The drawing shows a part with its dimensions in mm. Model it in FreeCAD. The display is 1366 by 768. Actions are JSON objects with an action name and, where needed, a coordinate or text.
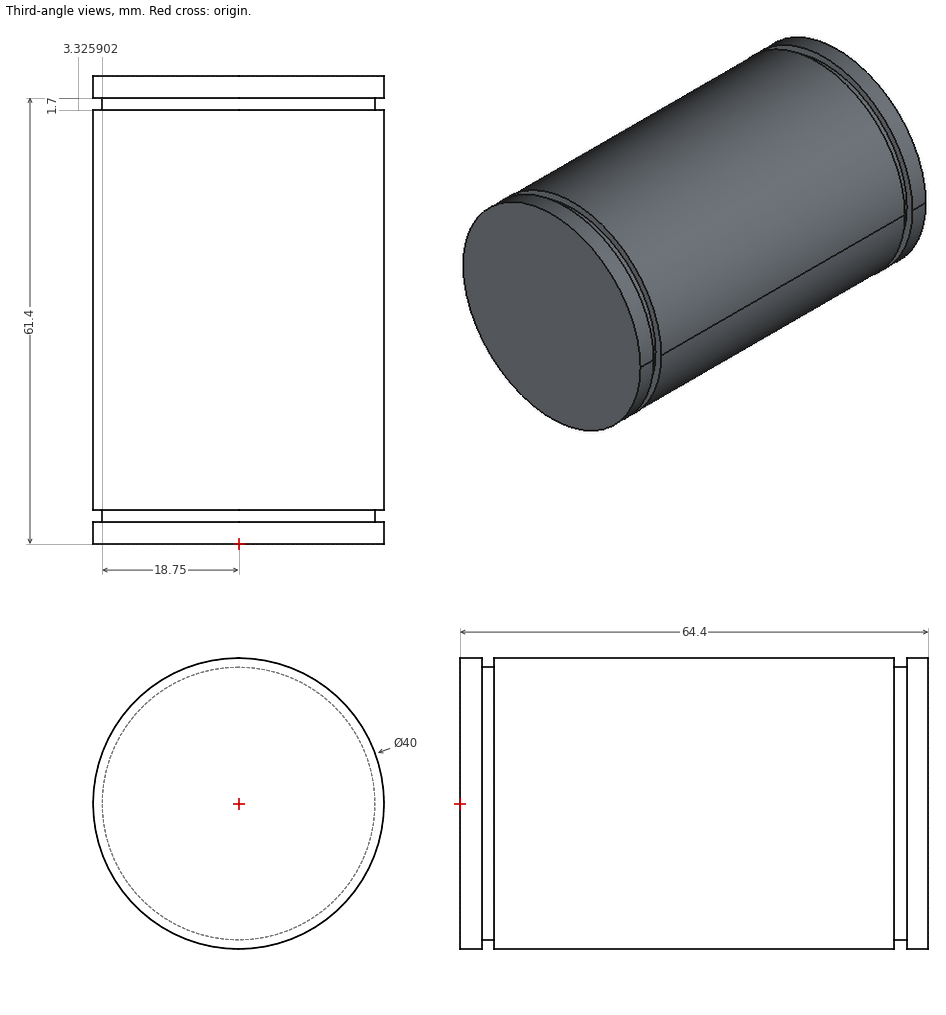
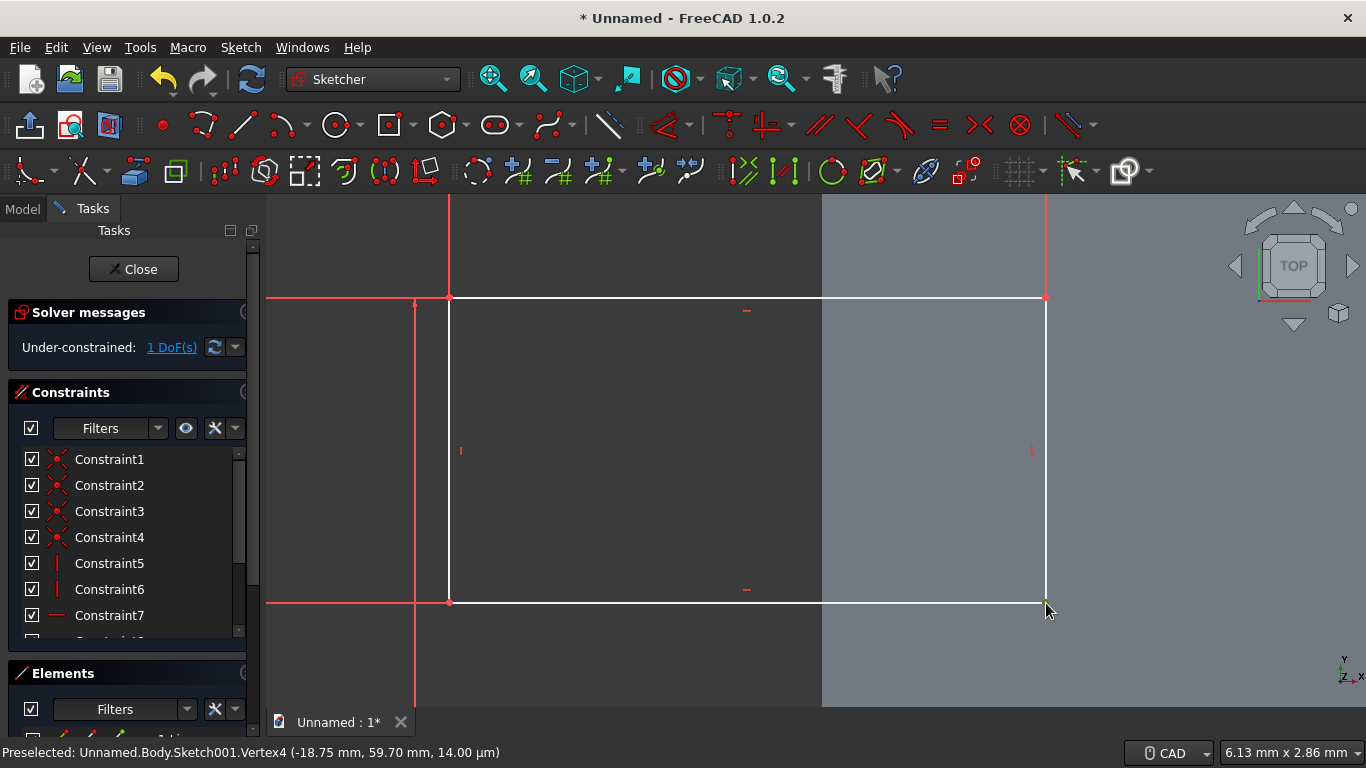
{"action": "left_click", "coordinate": [692, 126]}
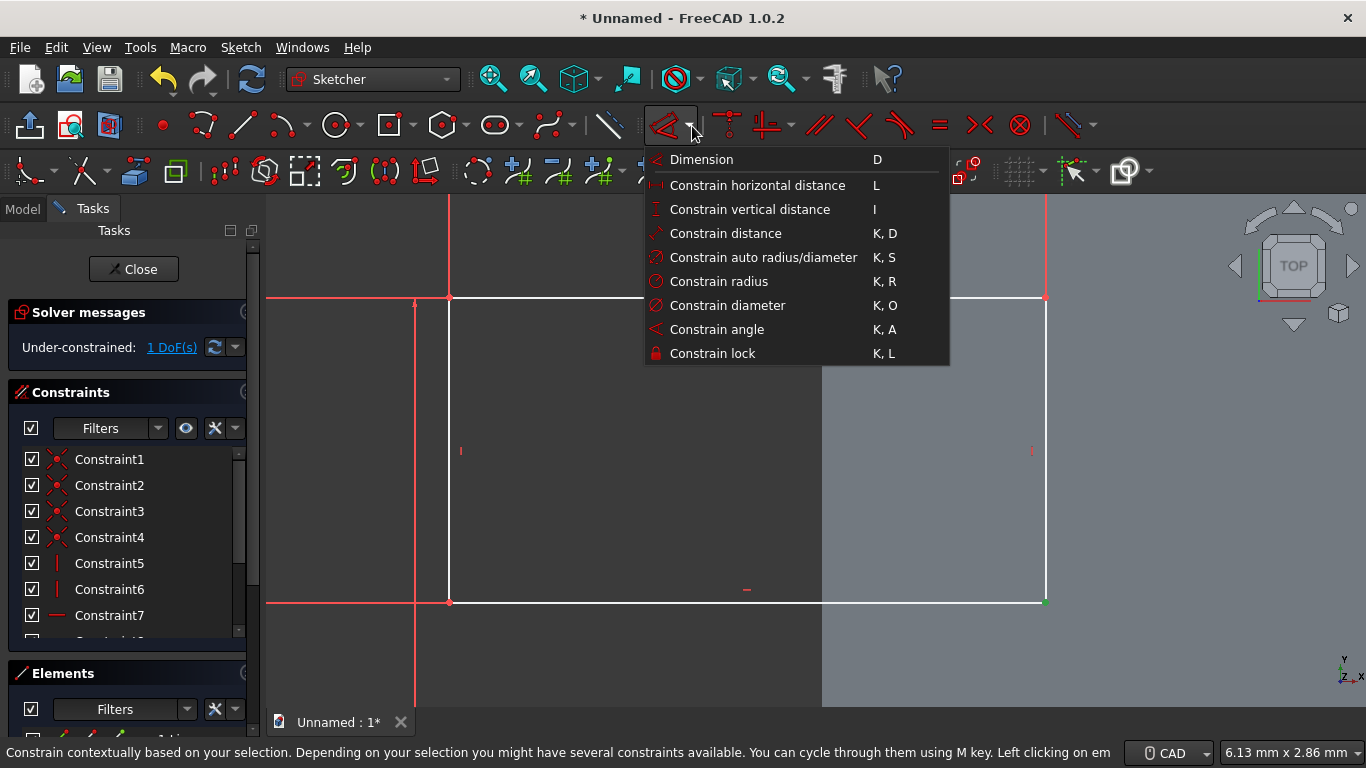
{"action": "left_click", "coordinate": [797, 185]}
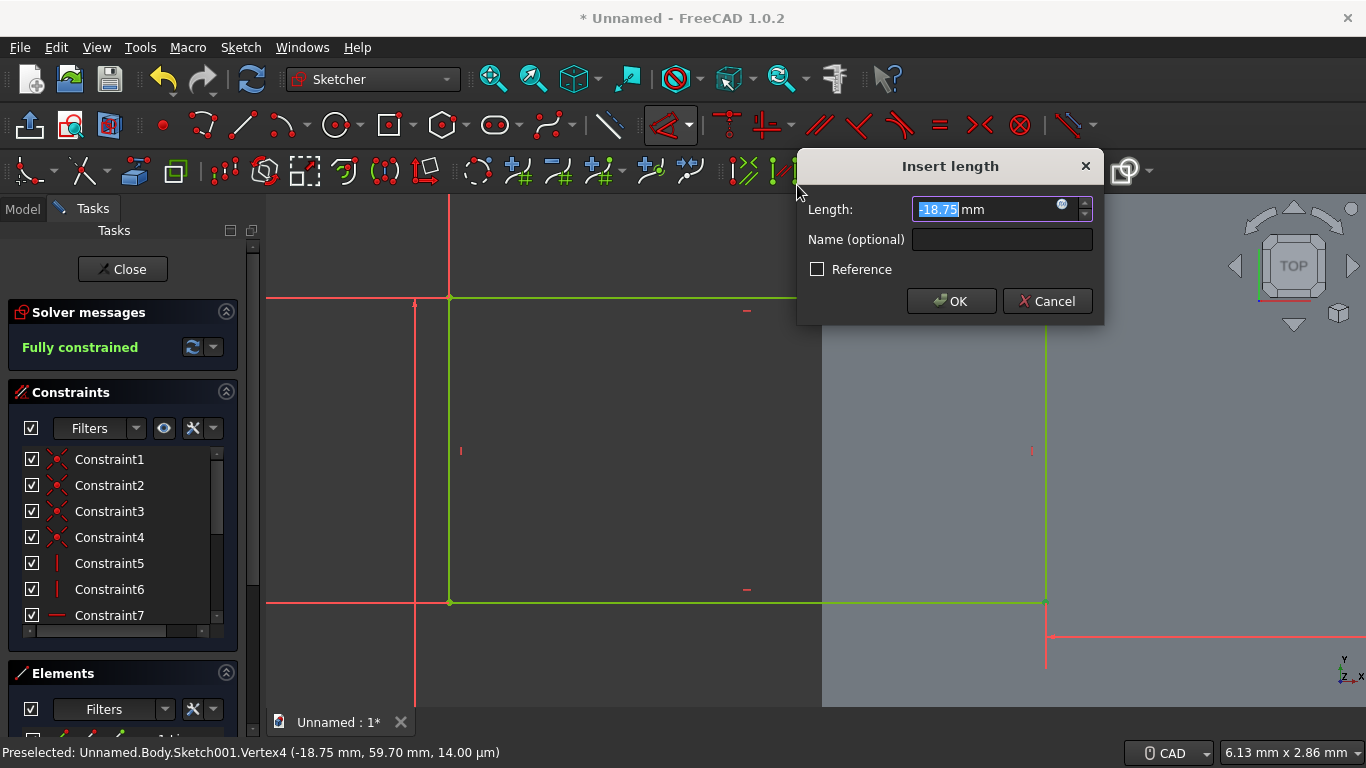
{"action": "type", "text": "-18.75"}
{"action": "key", "text": "Return"}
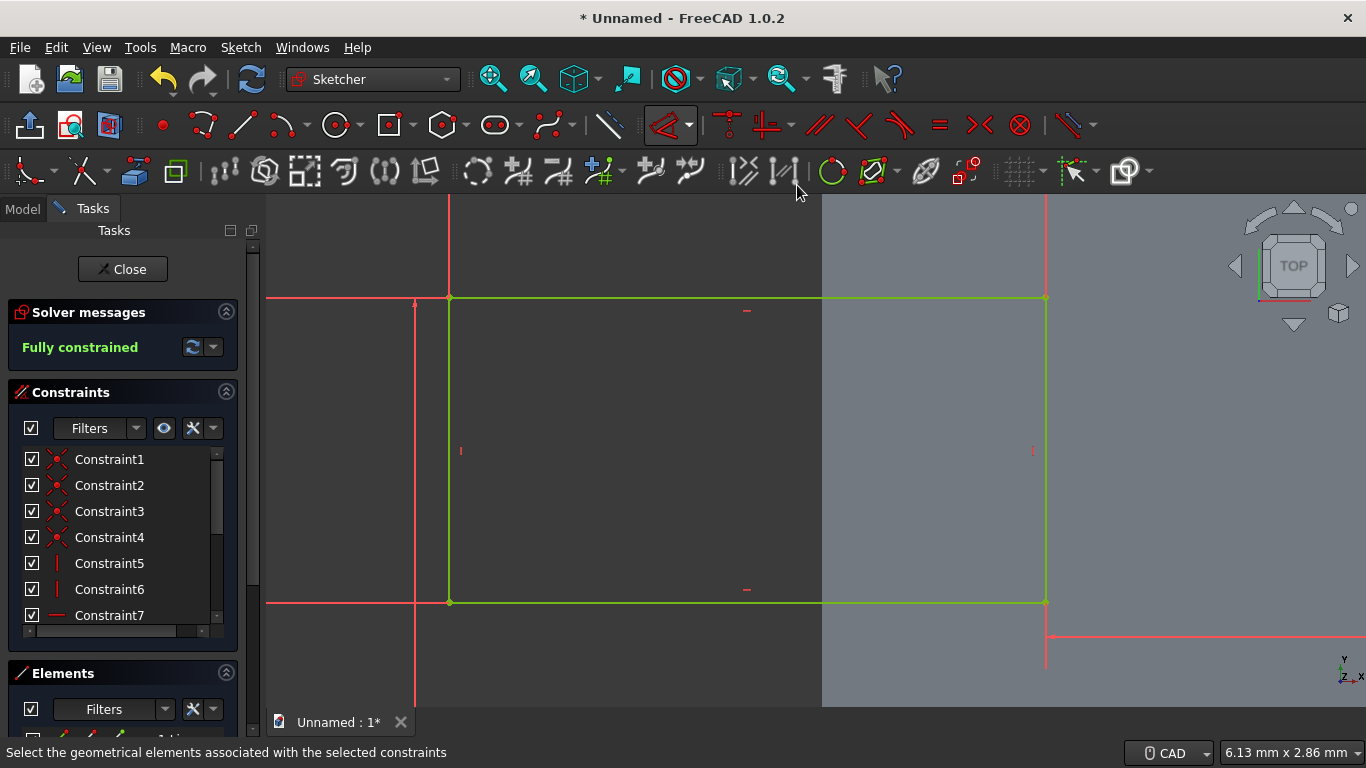
{"action": "left_click", "coordinate": [123, 269]}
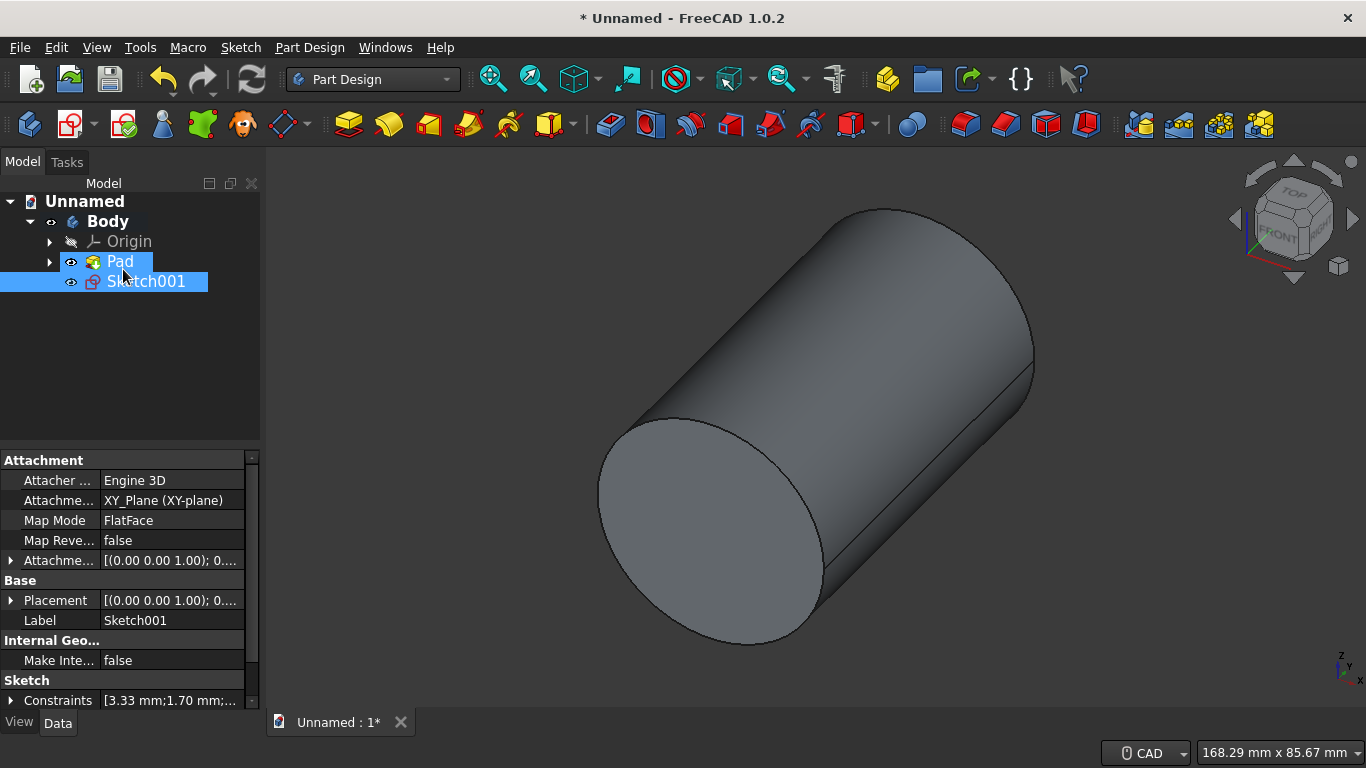
{"action": "left_click", "coordinate": [692, 124]}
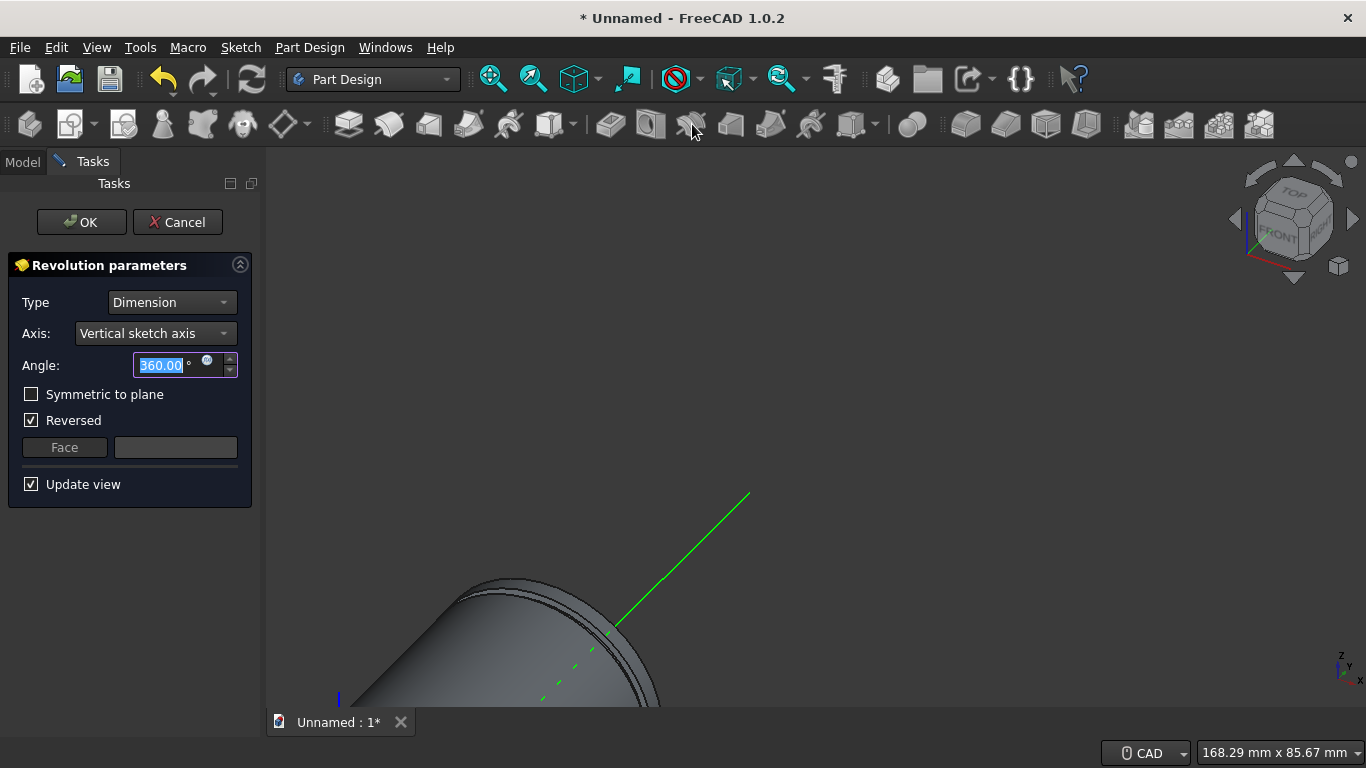
{"action": "left_click", "coordinate": [82, 222]}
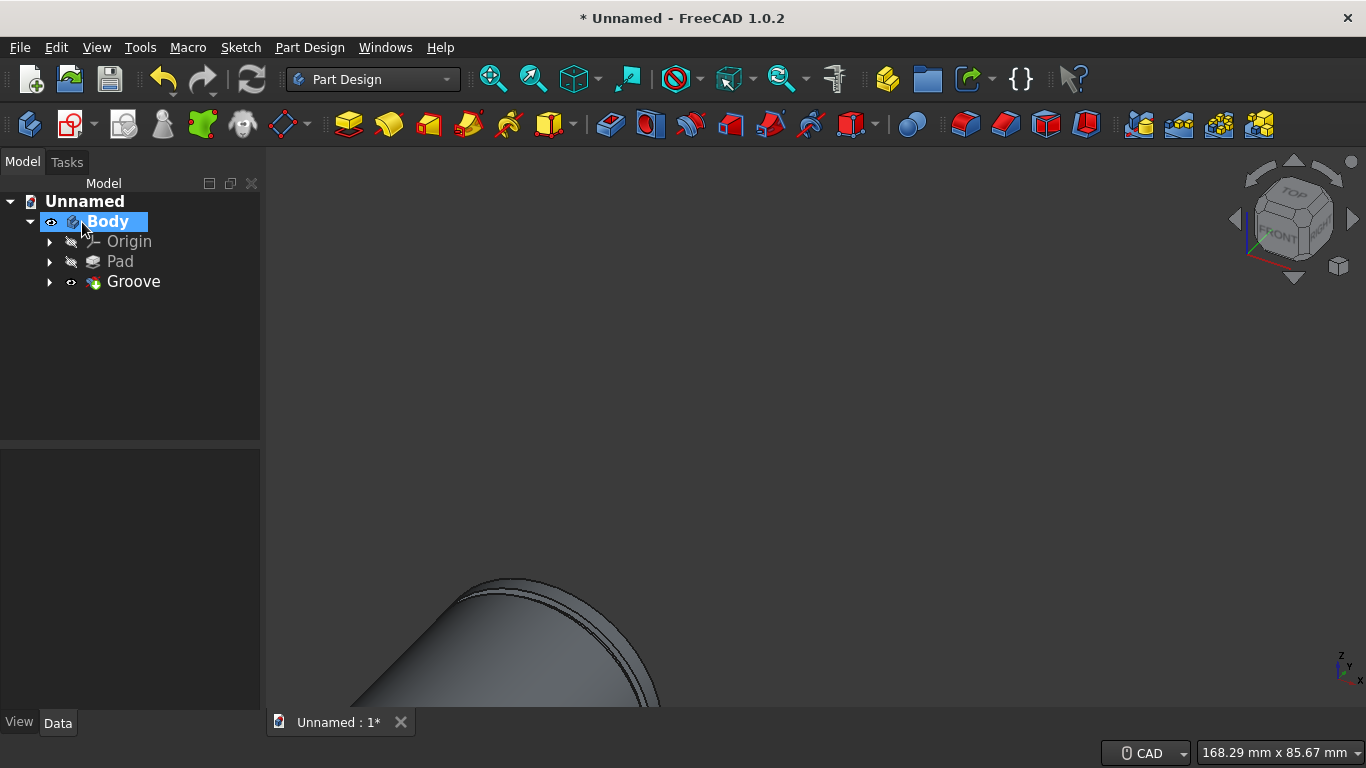
{"action": "left_click", "coordinate": [494, 80]}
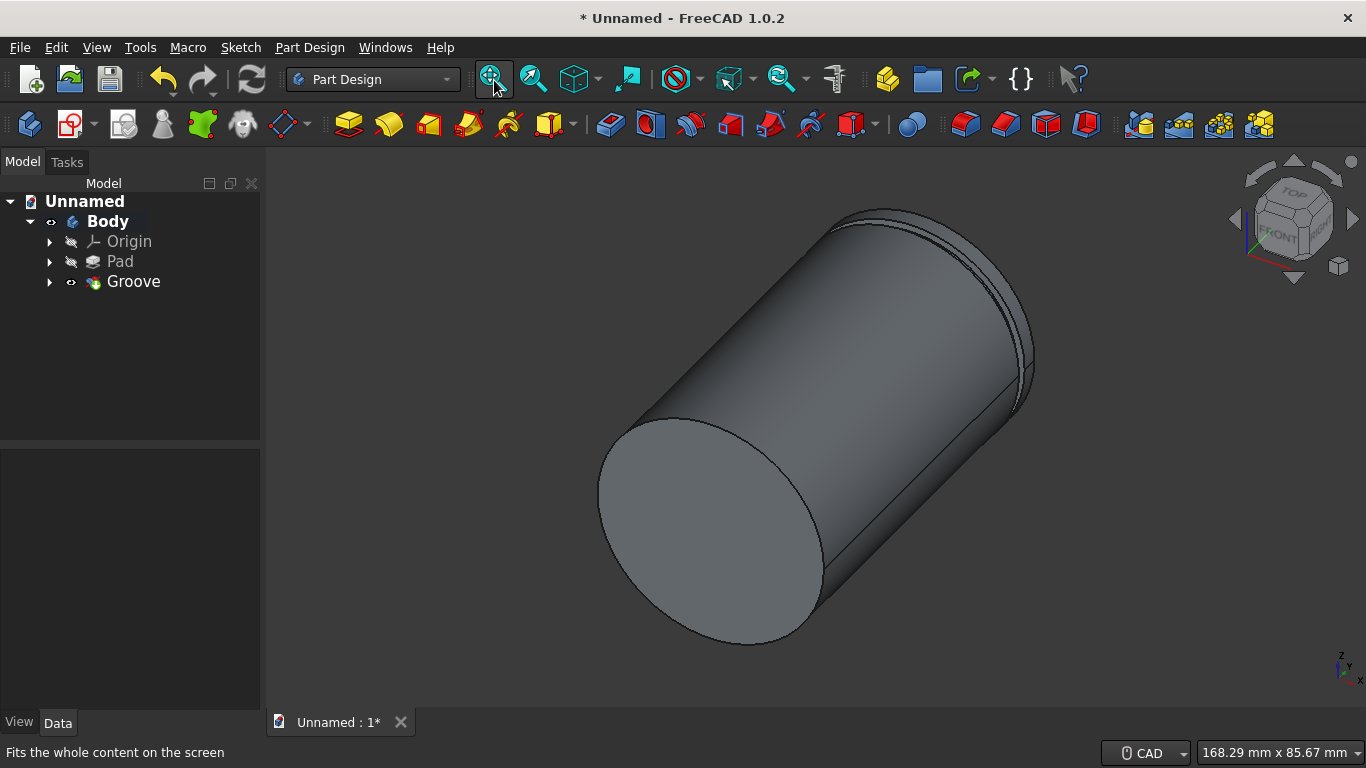
{"action": "left_click", "coordinate": [50, 242]}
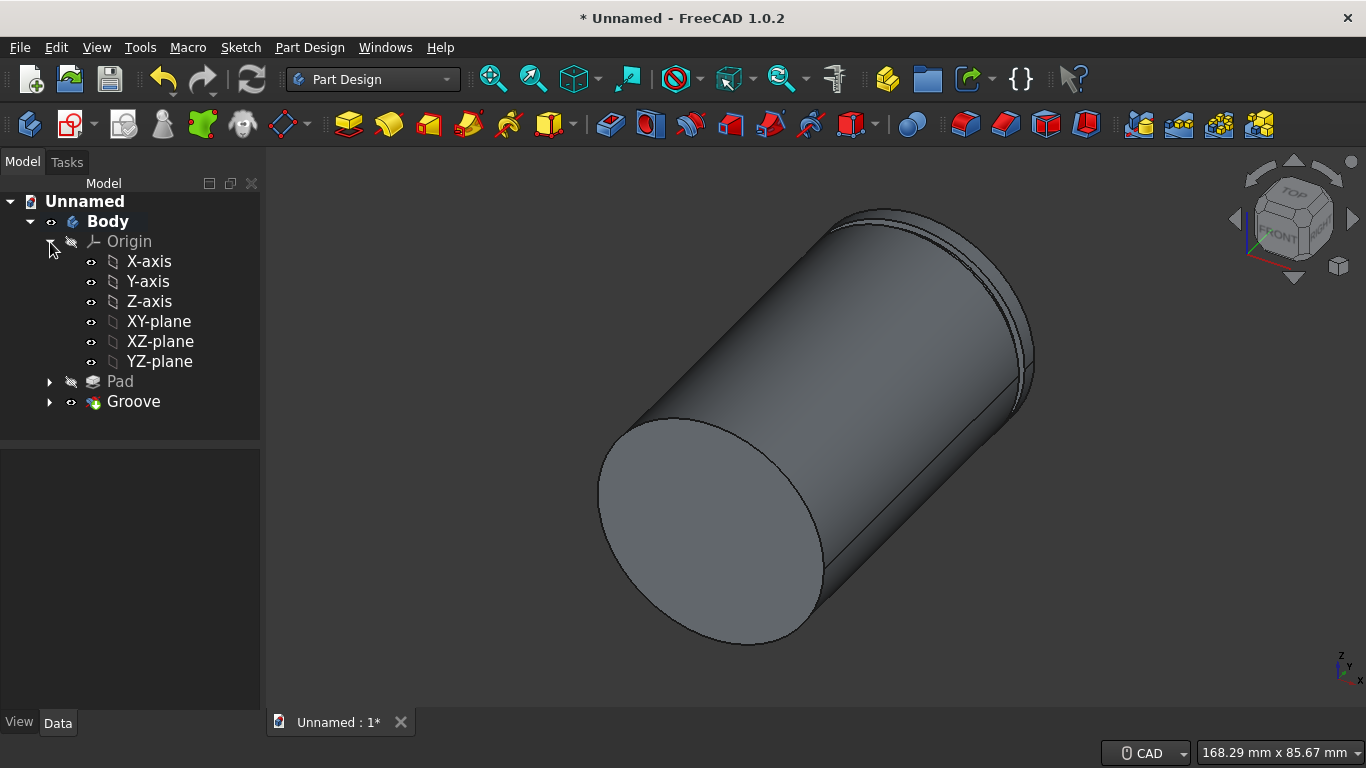
{"action": "left_click", "coordinate": [136, 342]}